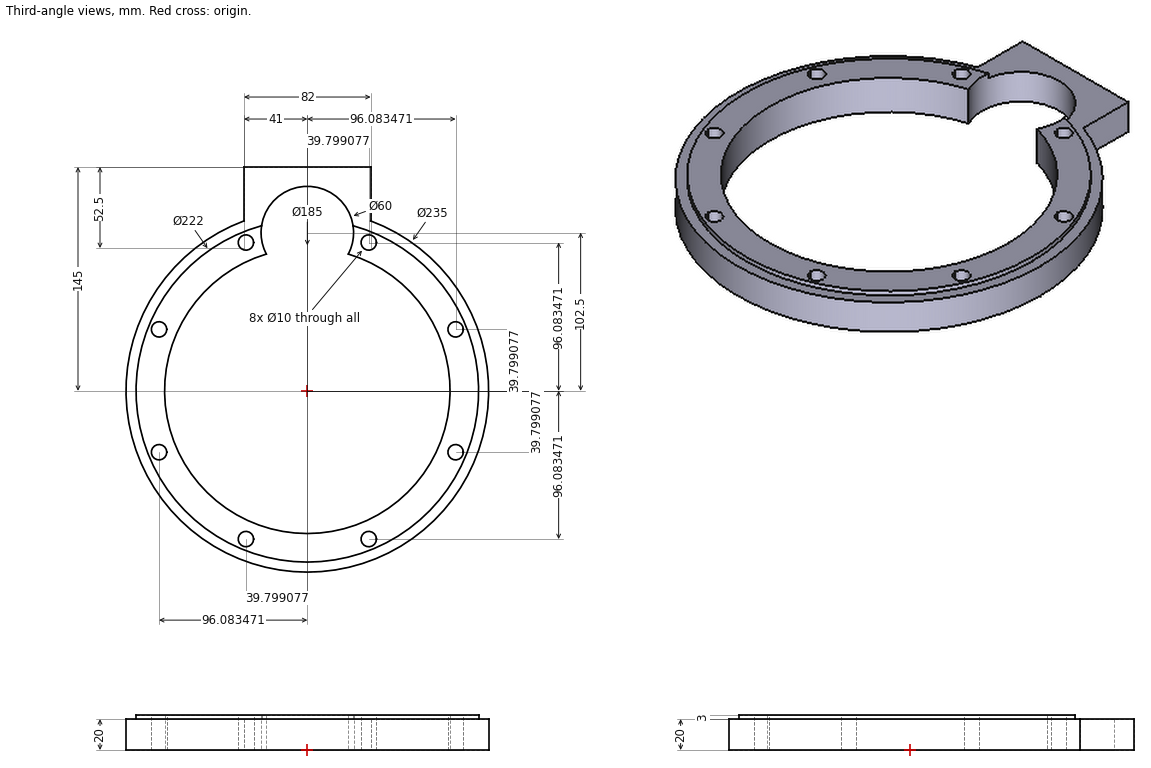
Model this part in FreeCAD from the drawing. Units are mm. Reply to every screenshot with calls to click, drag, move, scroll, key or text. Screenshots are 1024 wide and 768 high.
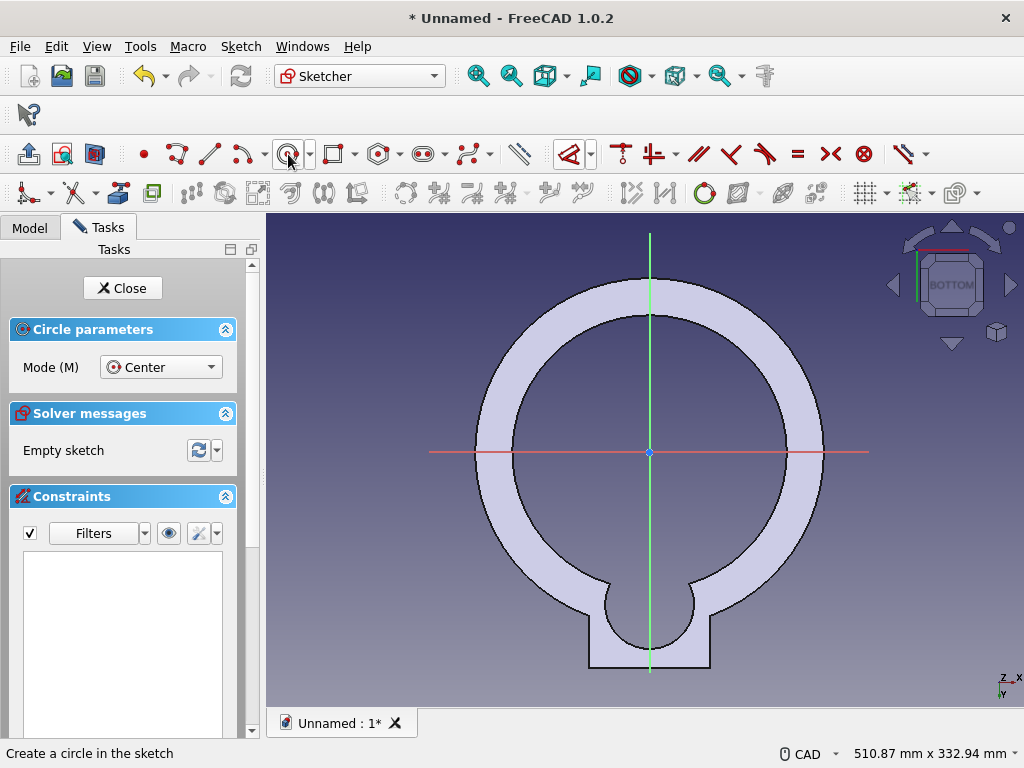
scroll(709, 595, up, 6)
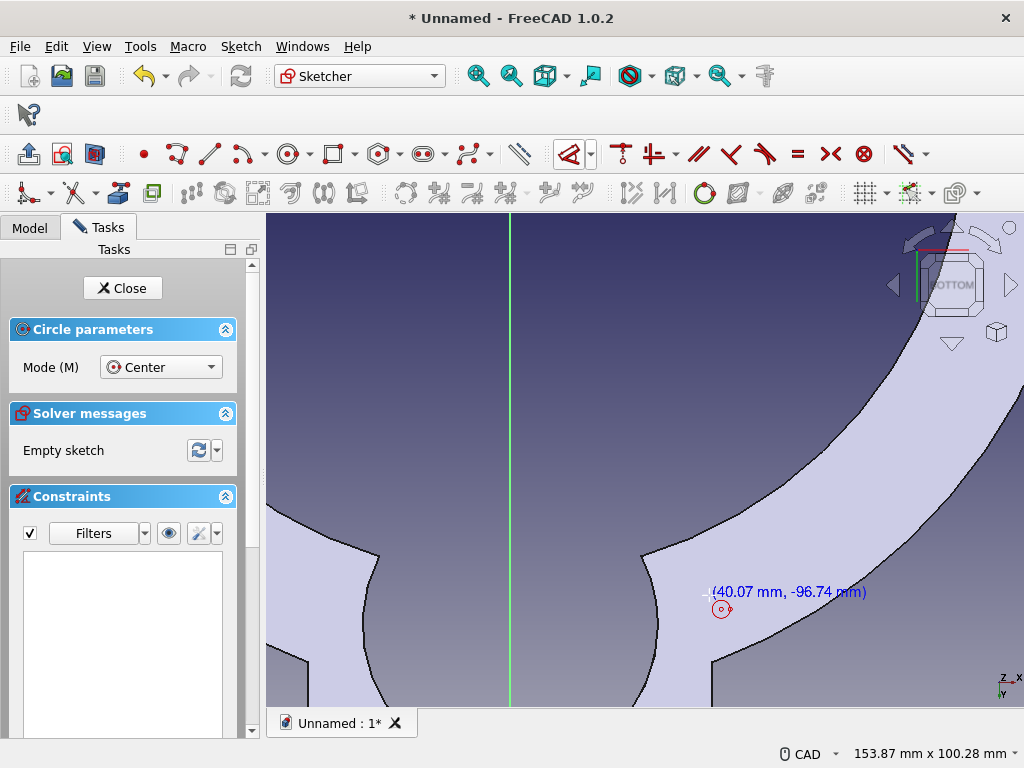
click(706, 593)
click(724, 576)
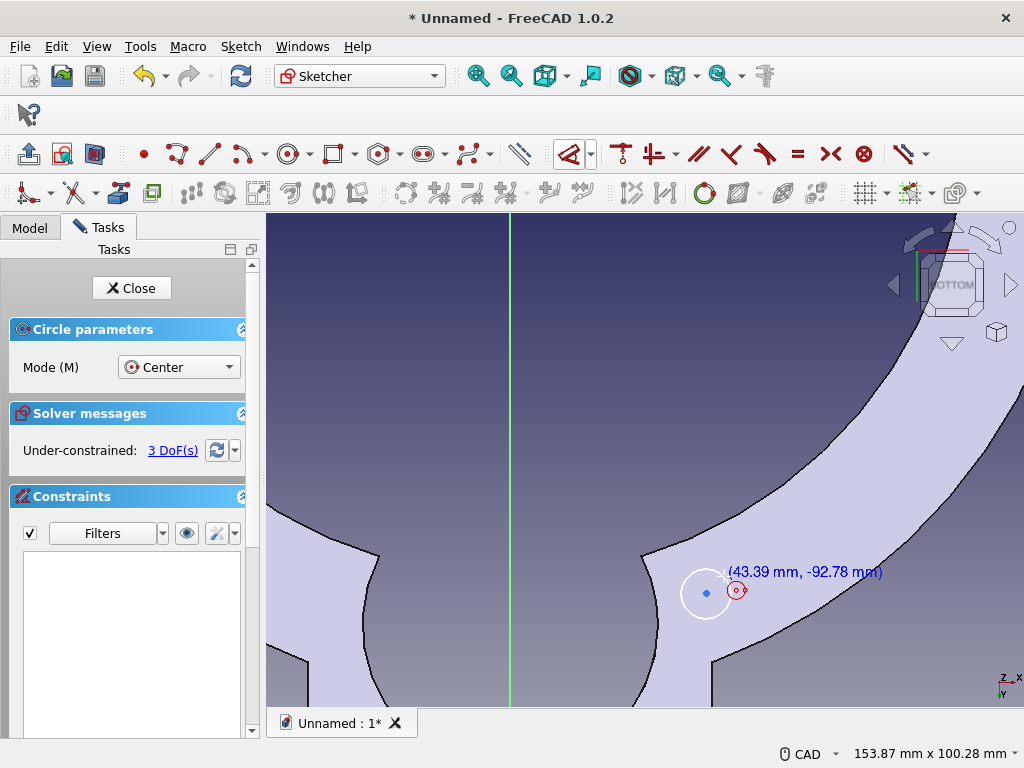
scroll(605, 607, down, 6)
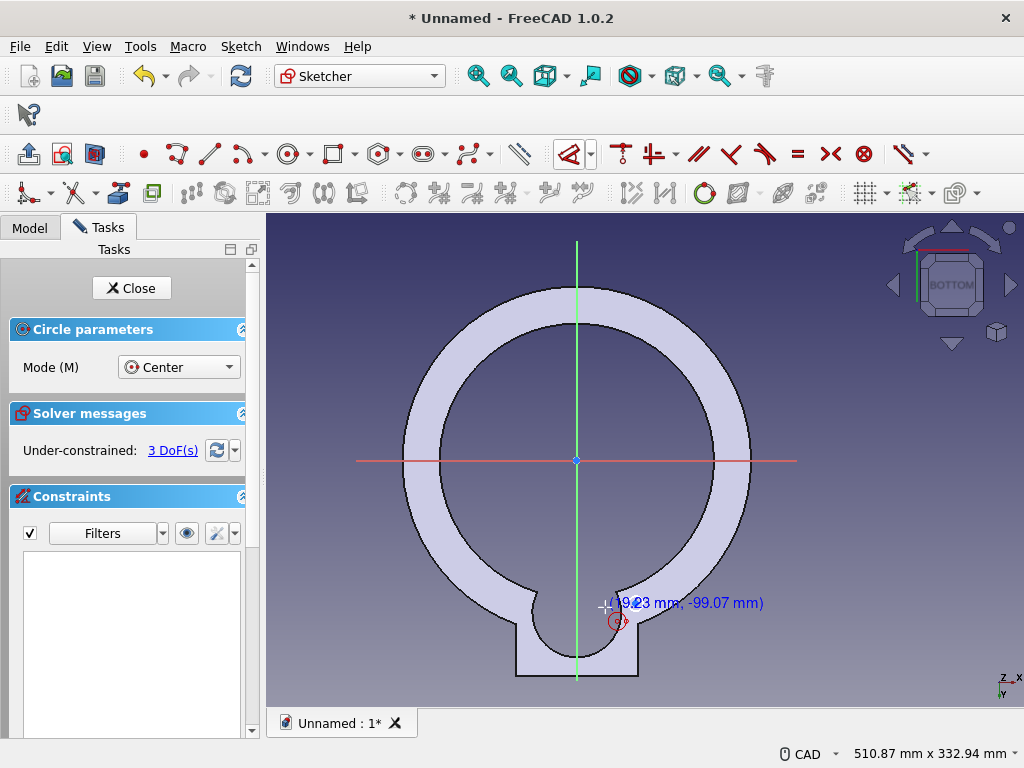
scroll(719, 520, up, 6)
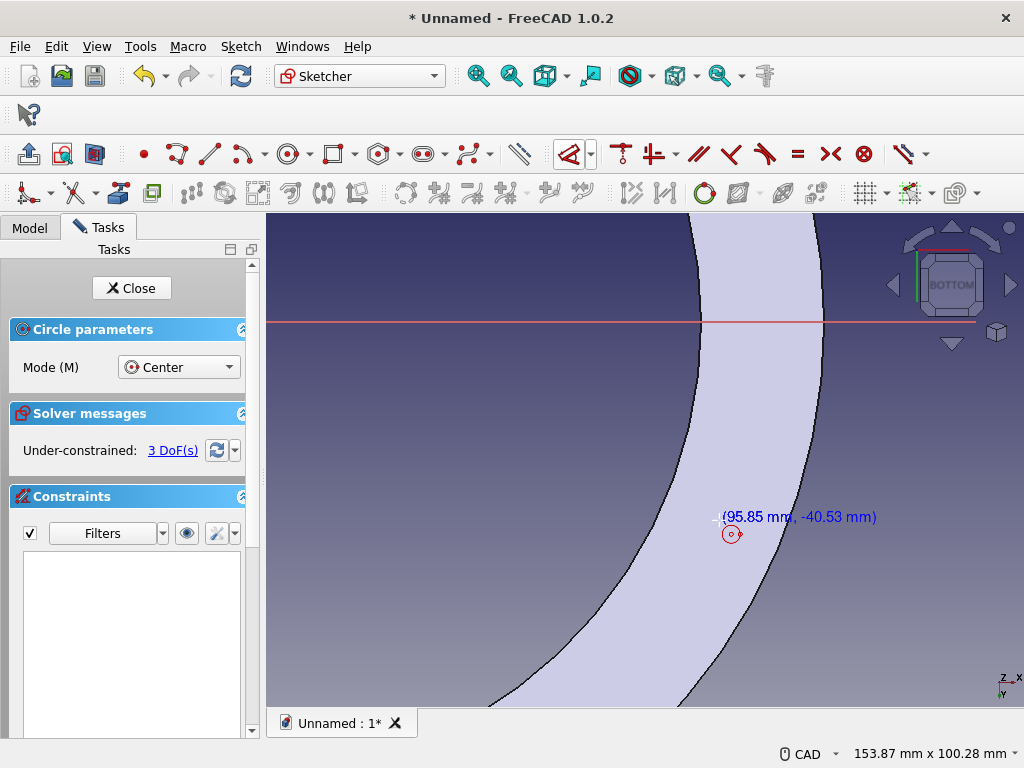
click(719, 518)
click(736, 501)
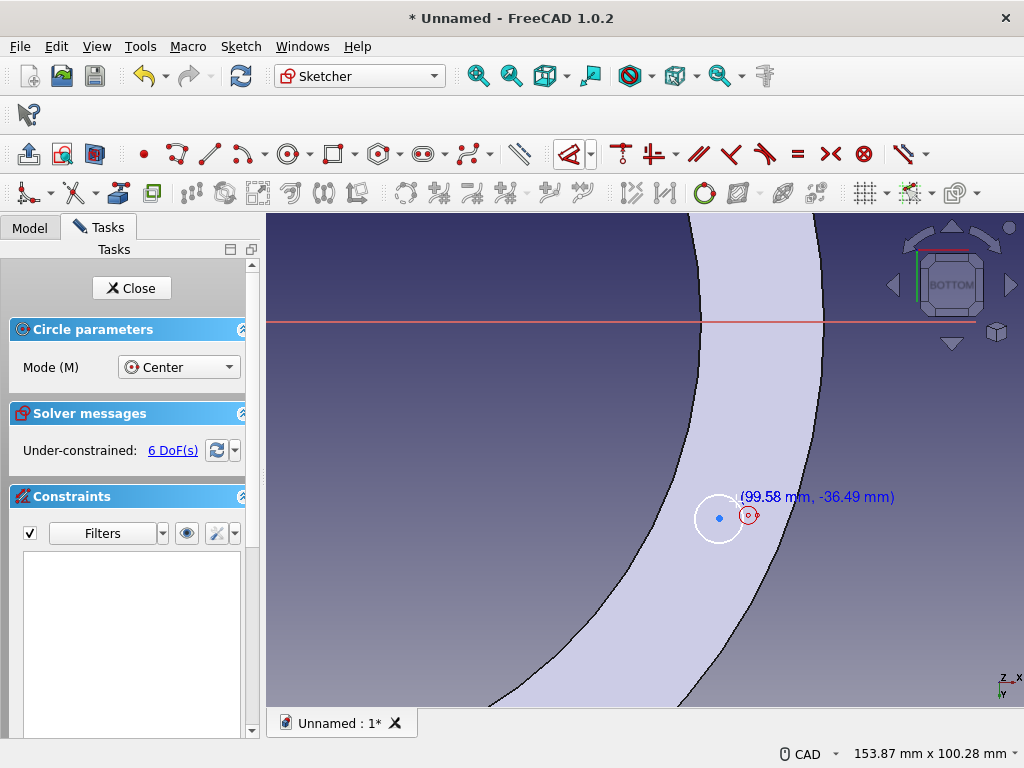
scroll(719, 519, down, 6)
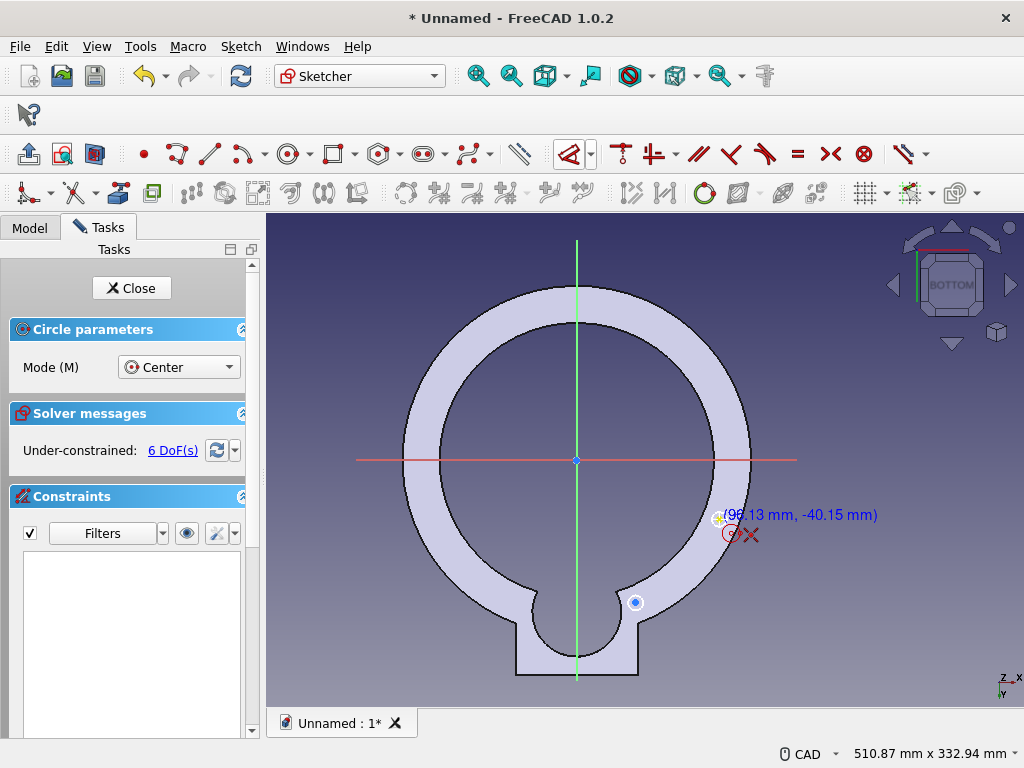
scroll(719, 401, up, 6)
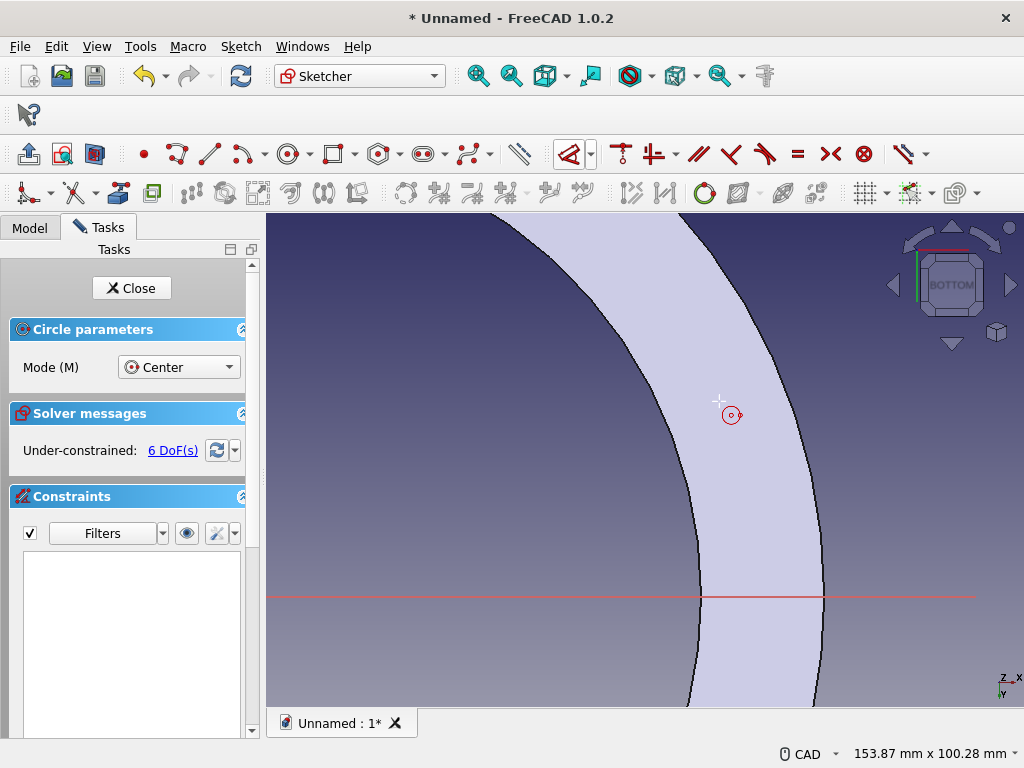
click(719, 400)
click(736, 383)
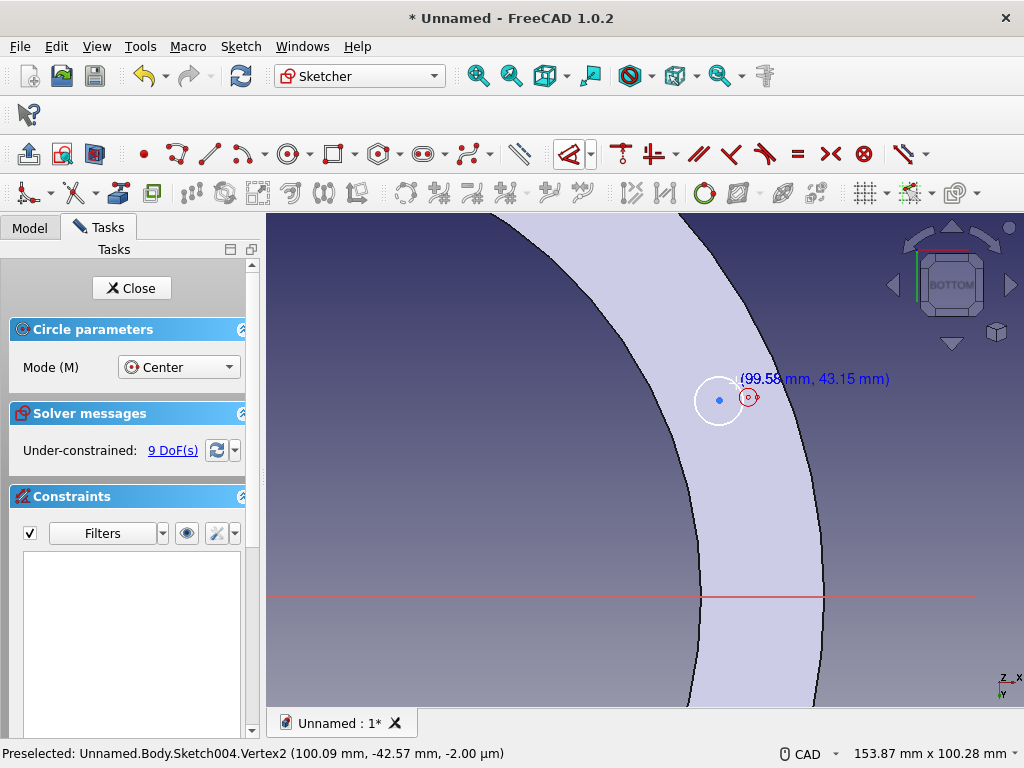
scroll(719, 401, down, 6)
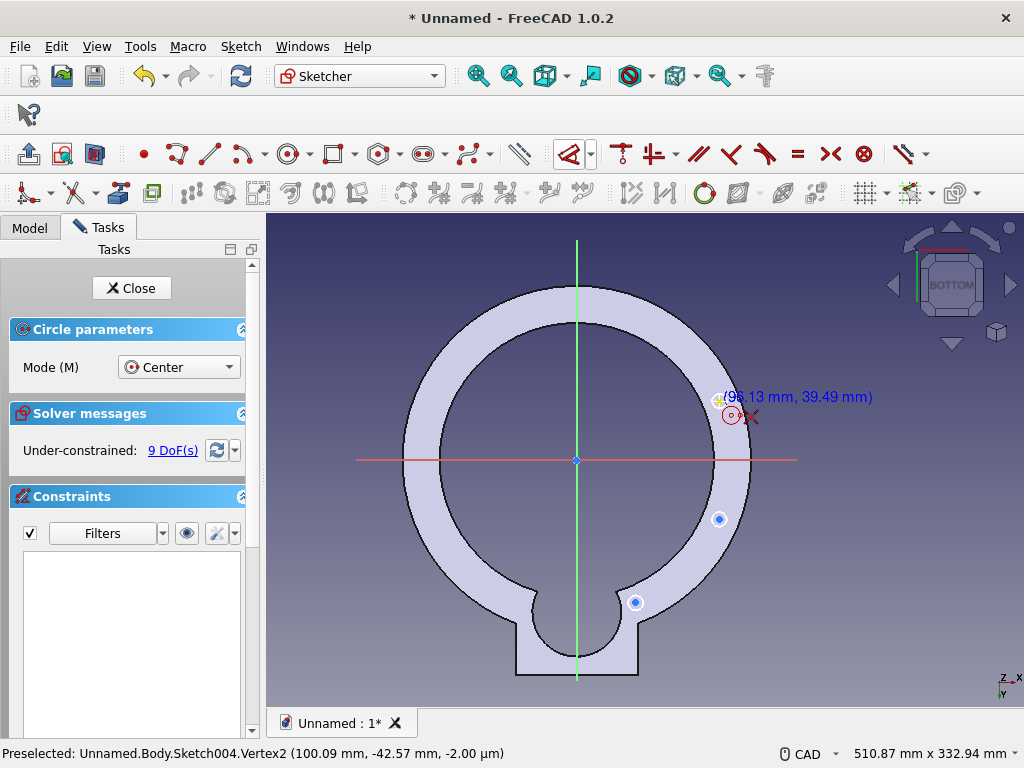
scroll(636, 318, up, 6)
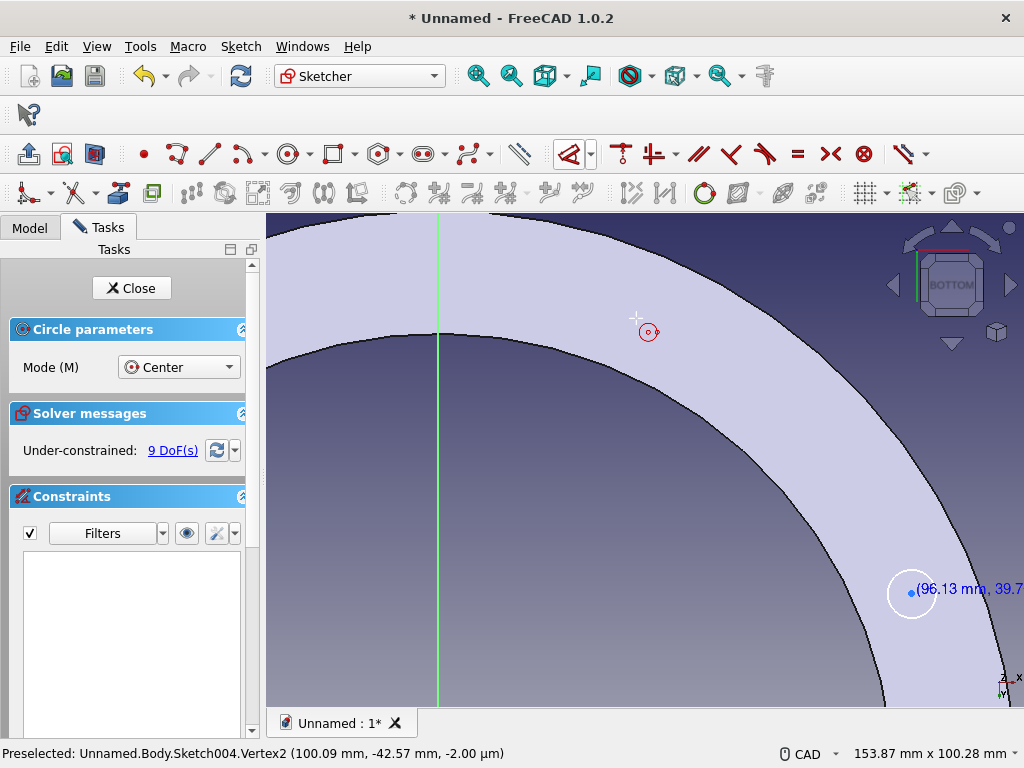
click(634, 316)
click(652, 299)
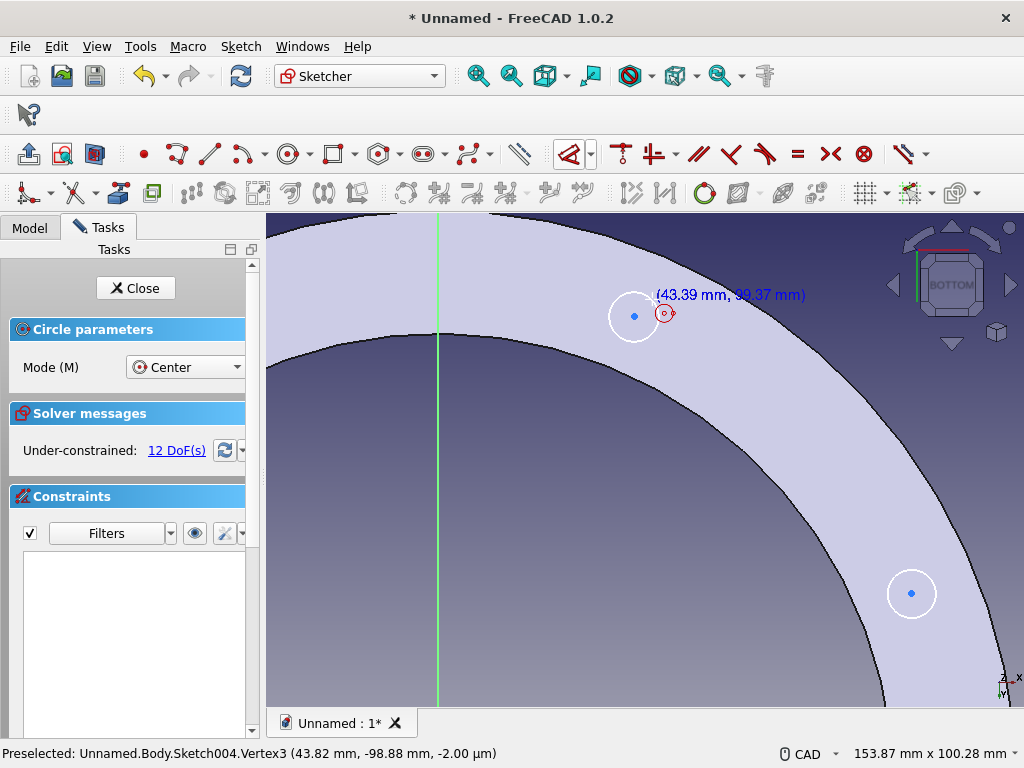
scroll(636, 318, down, 6)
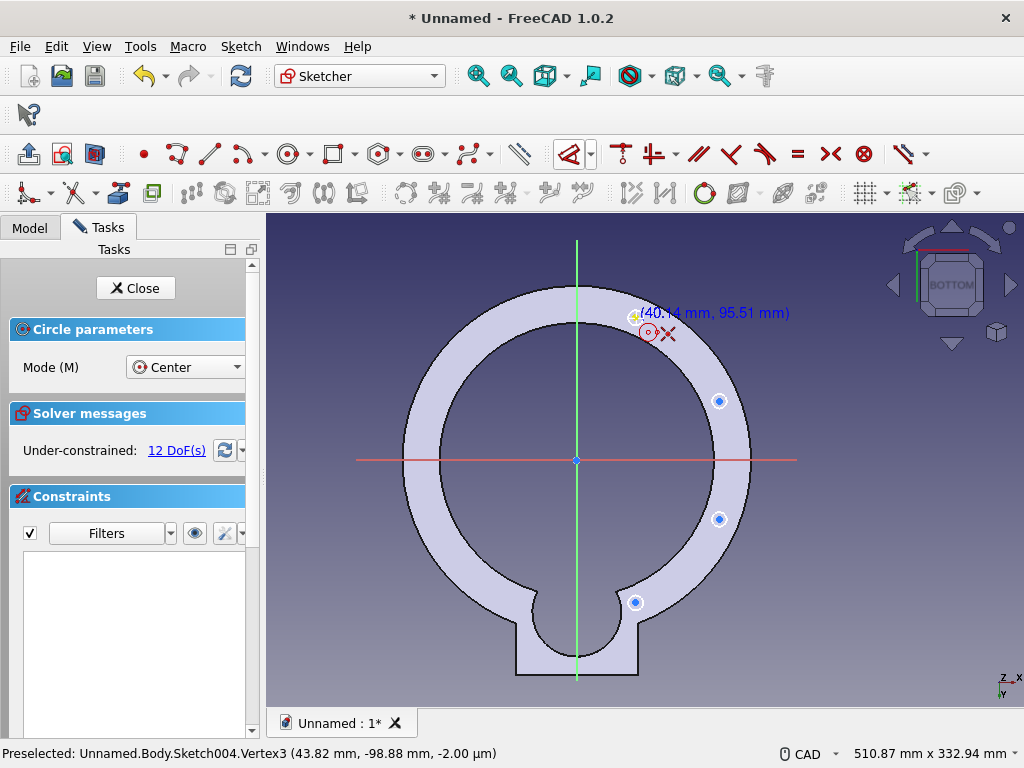
scroll(518, 318, up, 6)